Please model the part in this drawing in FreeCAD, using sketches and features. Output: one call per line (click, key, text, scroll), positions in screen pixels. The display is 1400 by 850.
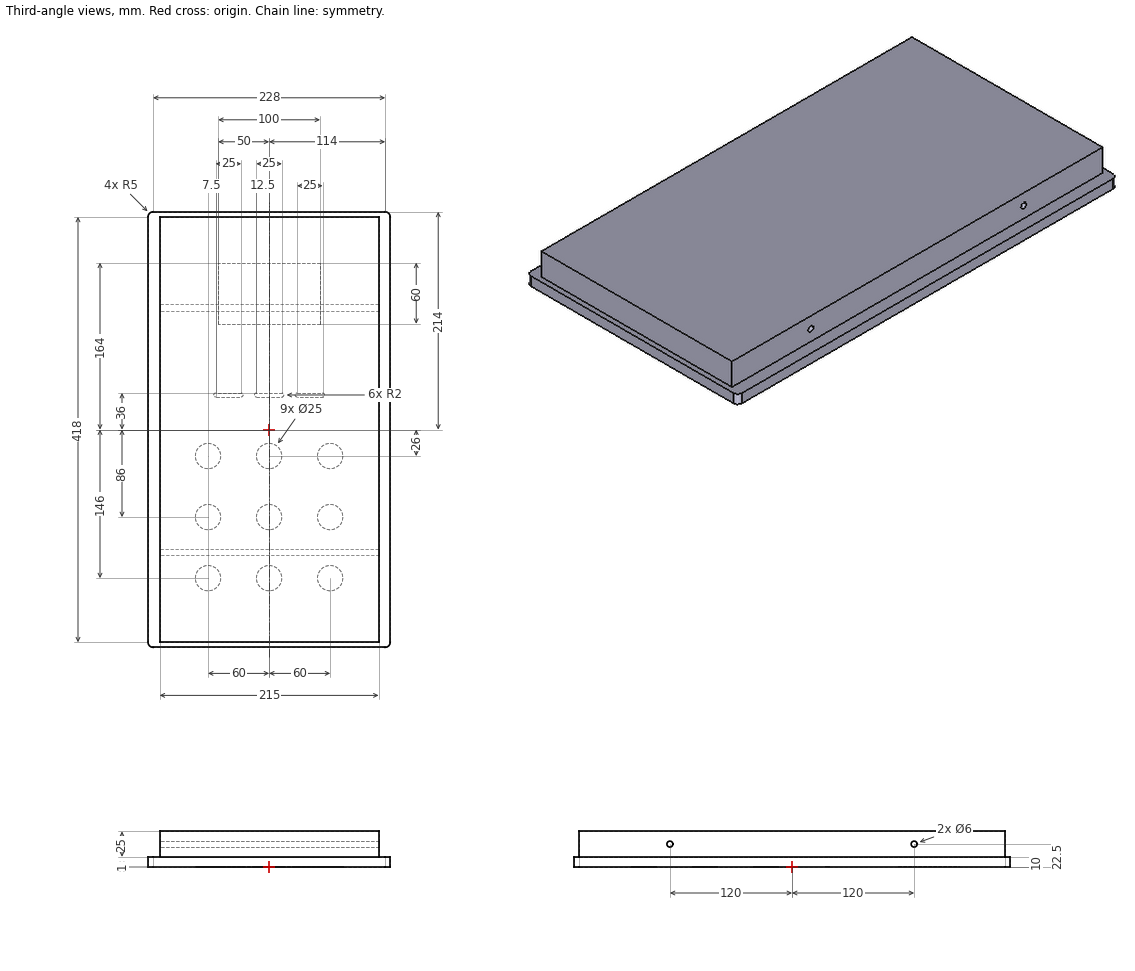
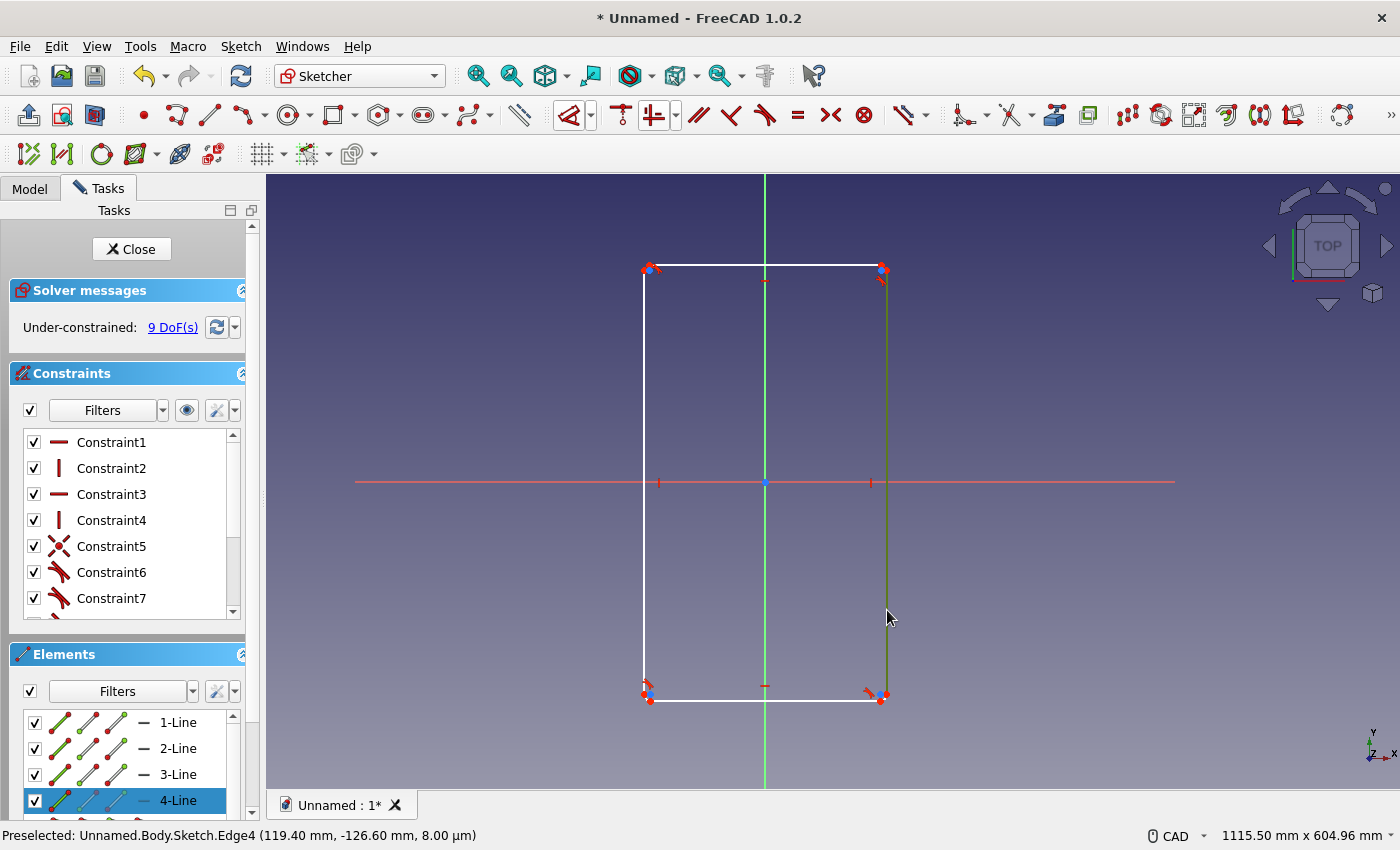
scroll(885, 267, up, 7)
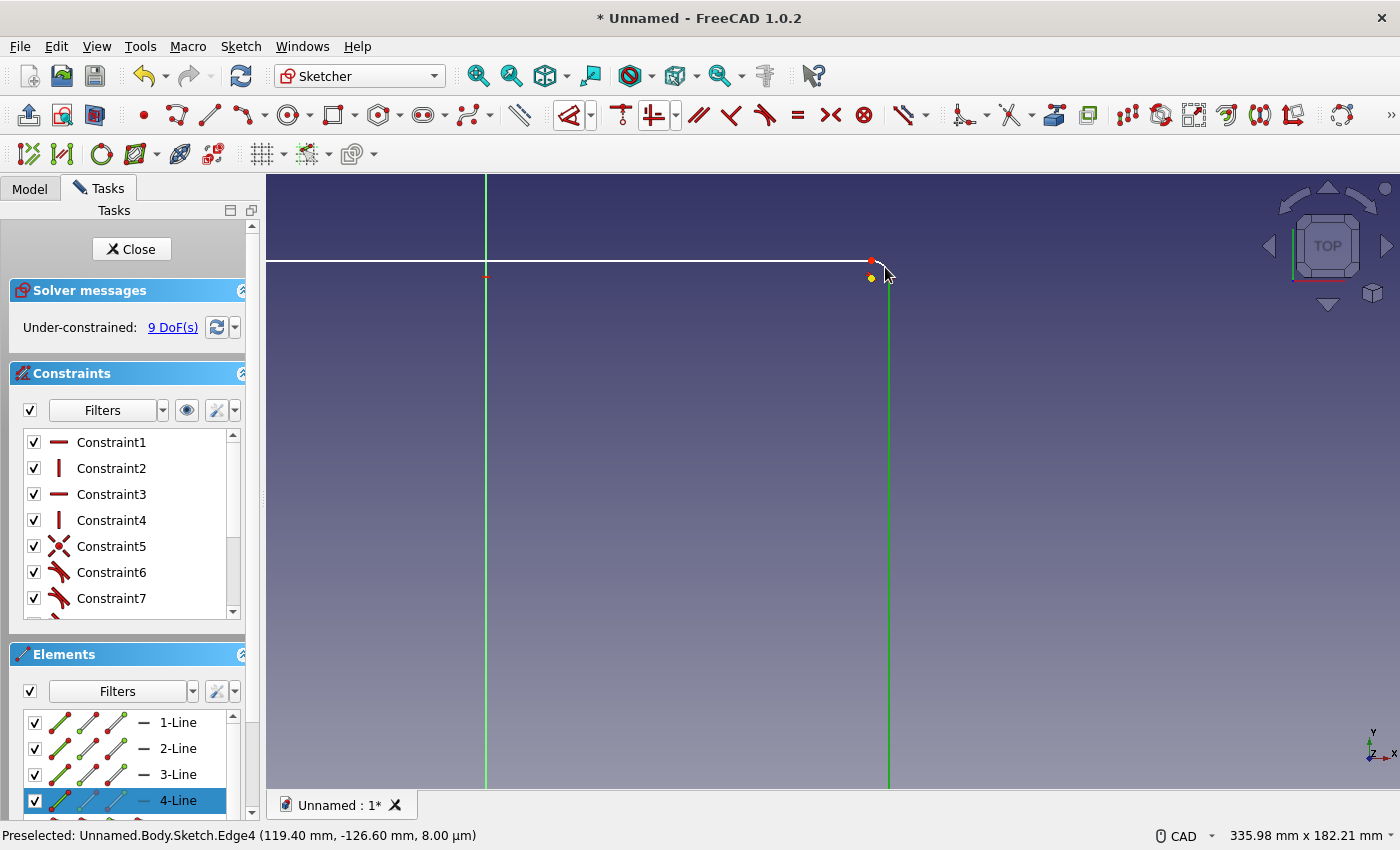
click(884, 266)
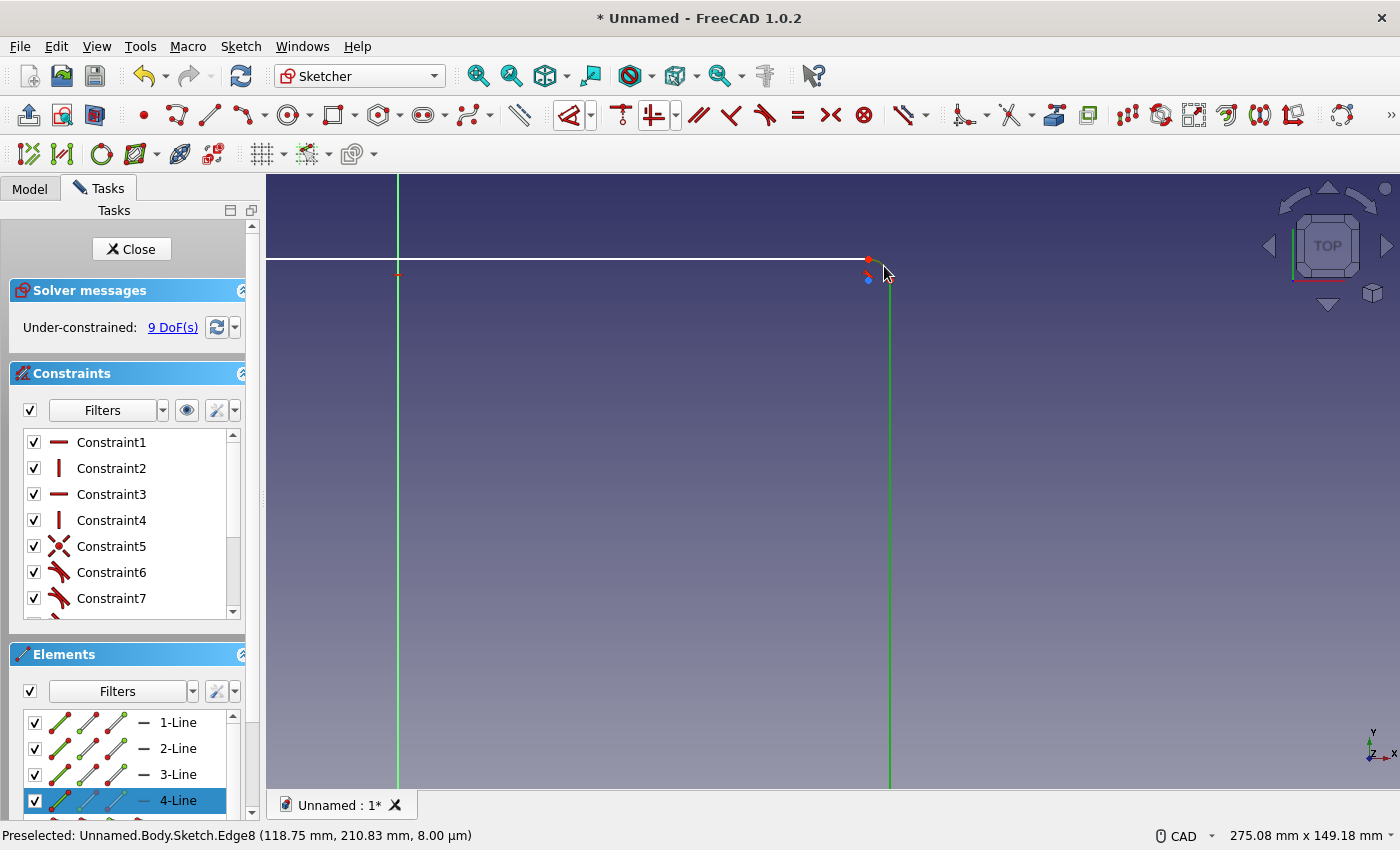
click(765, 116)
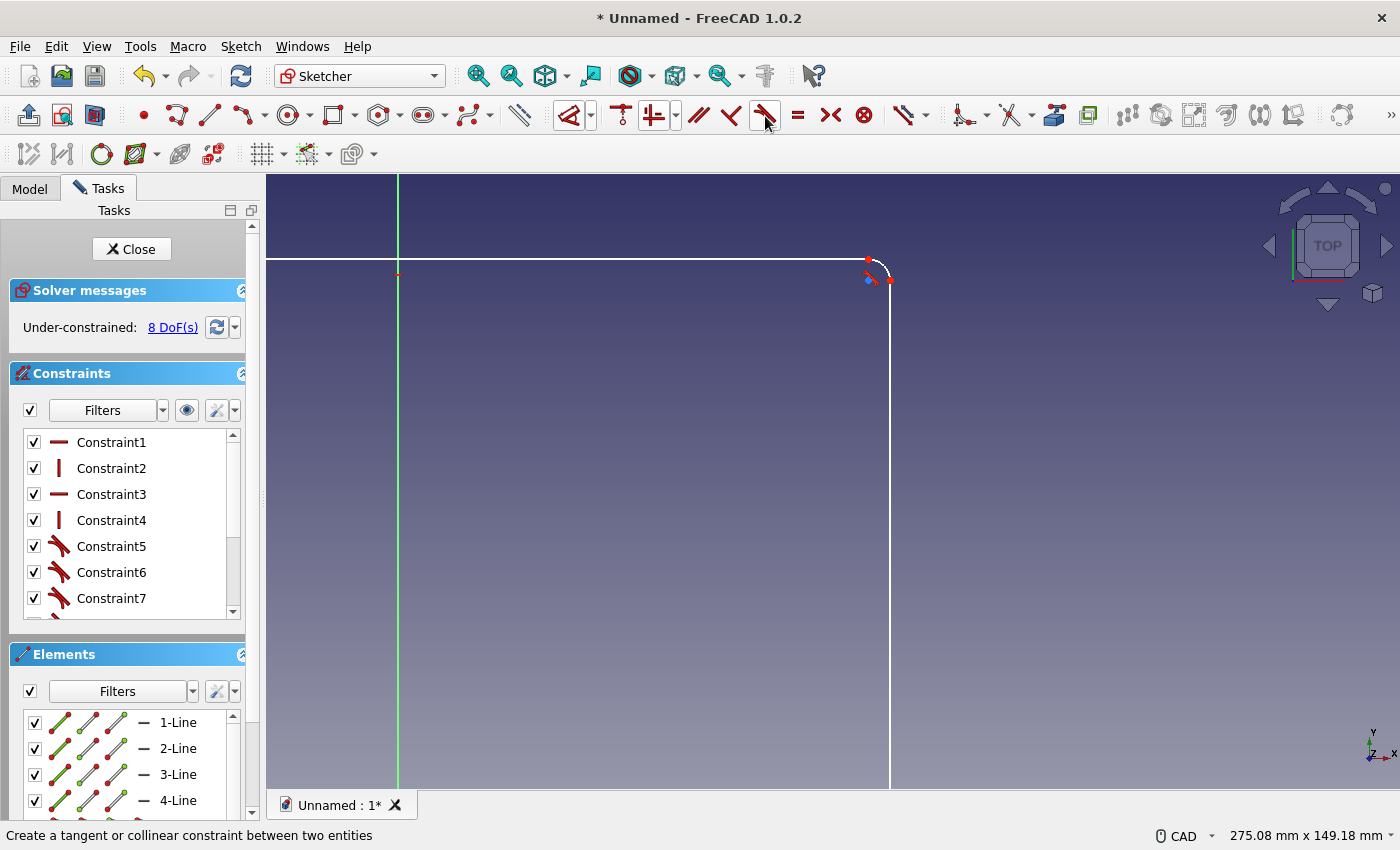
scroll(885, 266, down, 7)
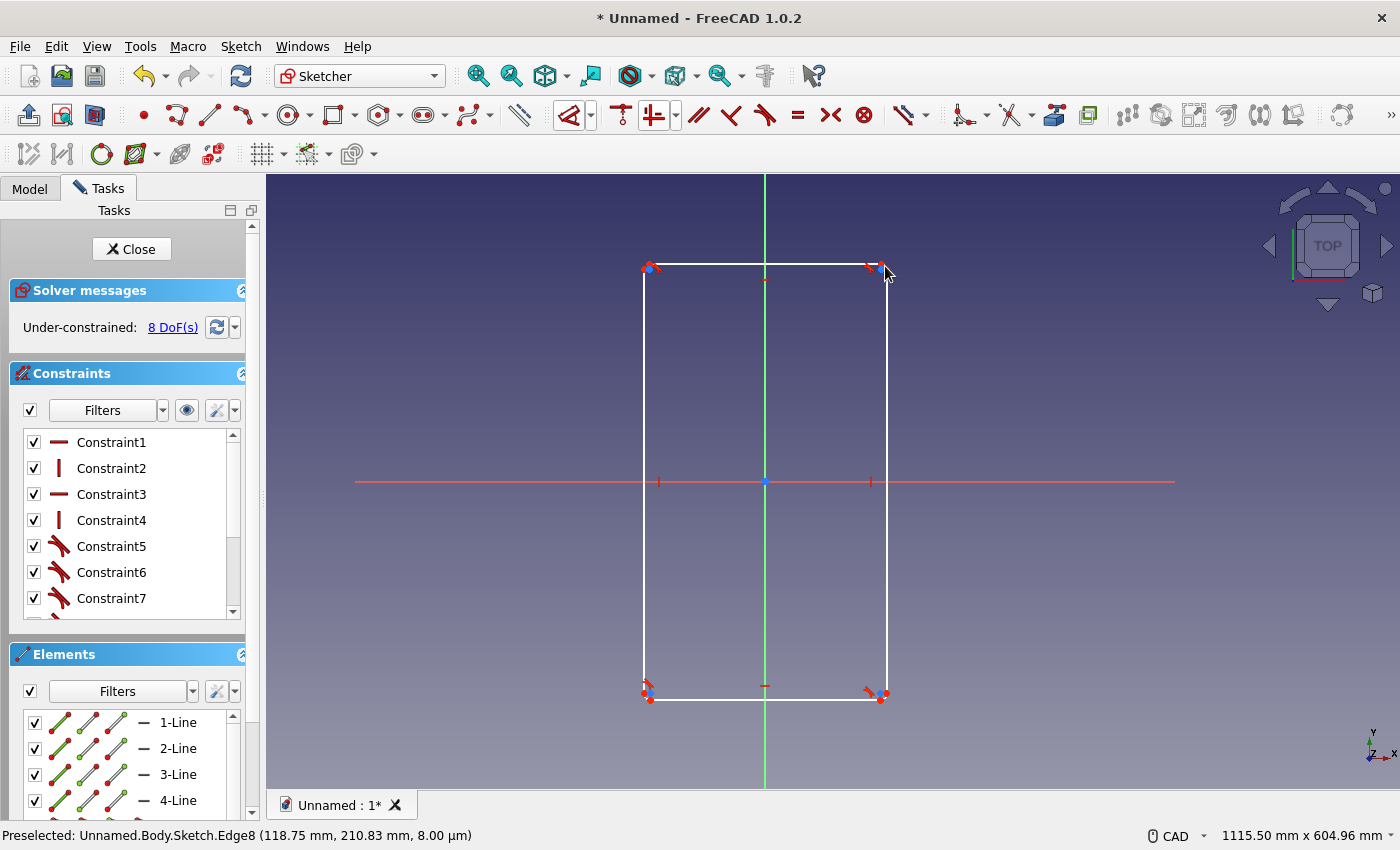
scroll(647, 265, up, 9)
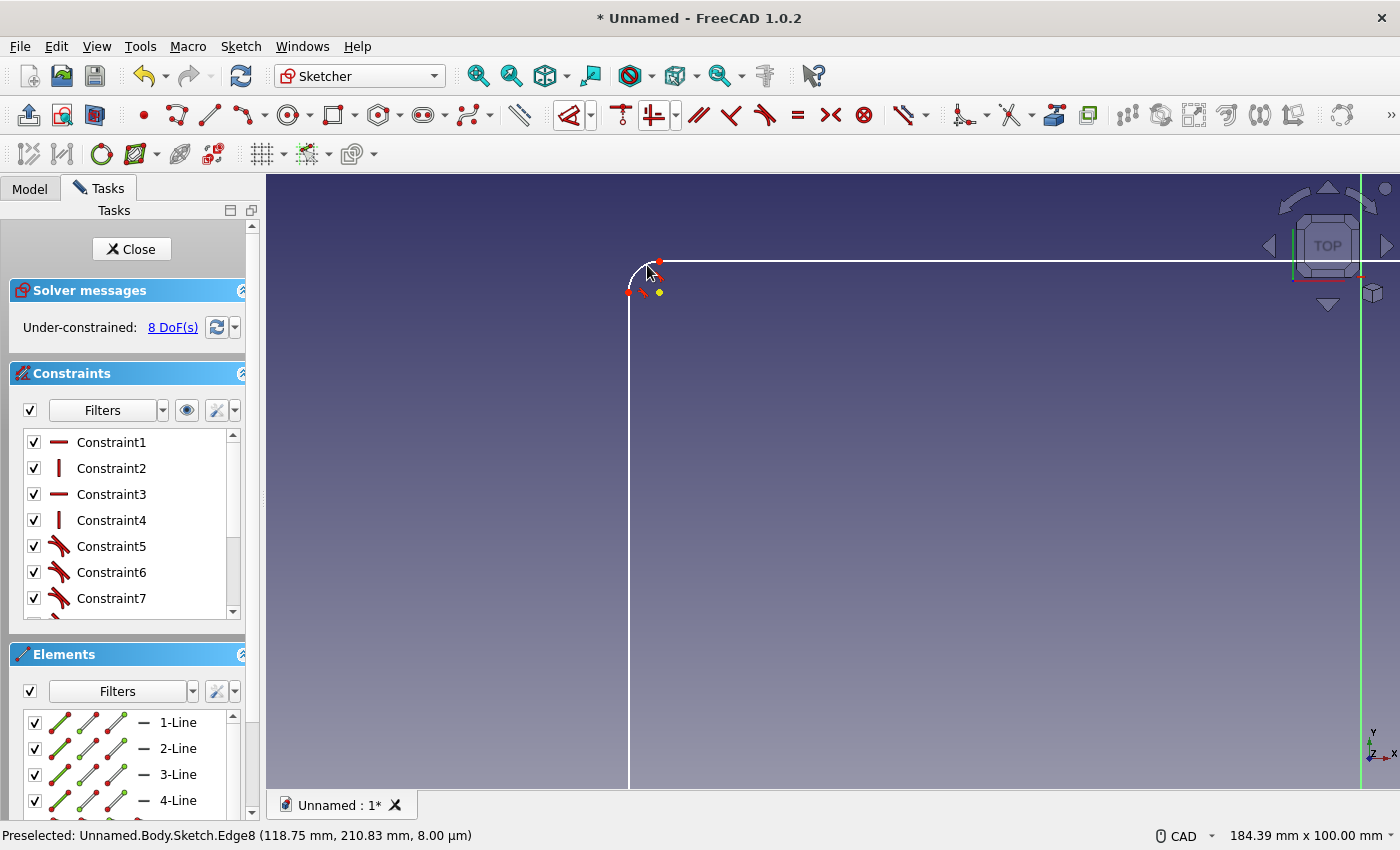
click(646, 265)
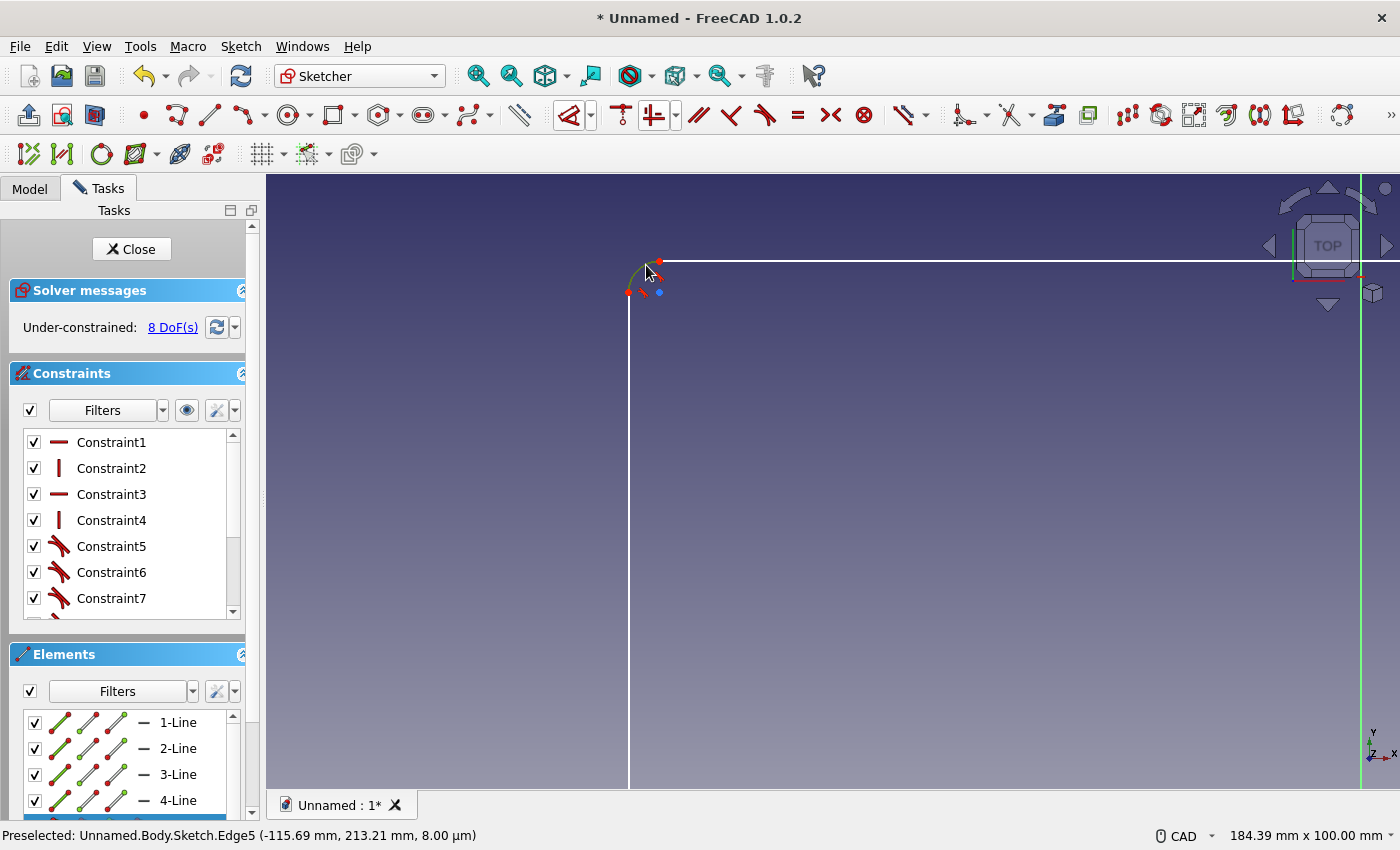
scroll(646, 265, down, 9)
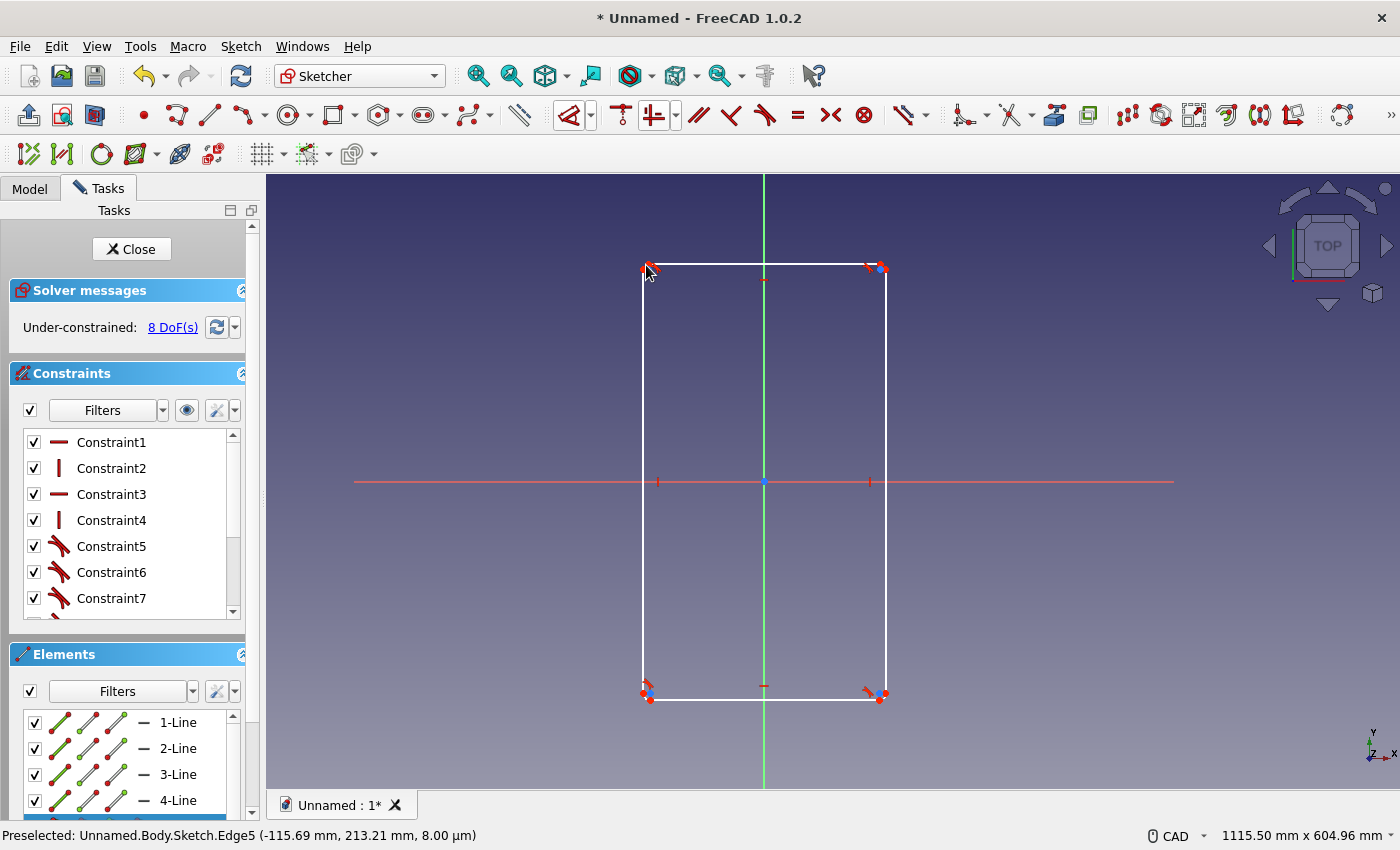
scroll(644, 697, up, 8)